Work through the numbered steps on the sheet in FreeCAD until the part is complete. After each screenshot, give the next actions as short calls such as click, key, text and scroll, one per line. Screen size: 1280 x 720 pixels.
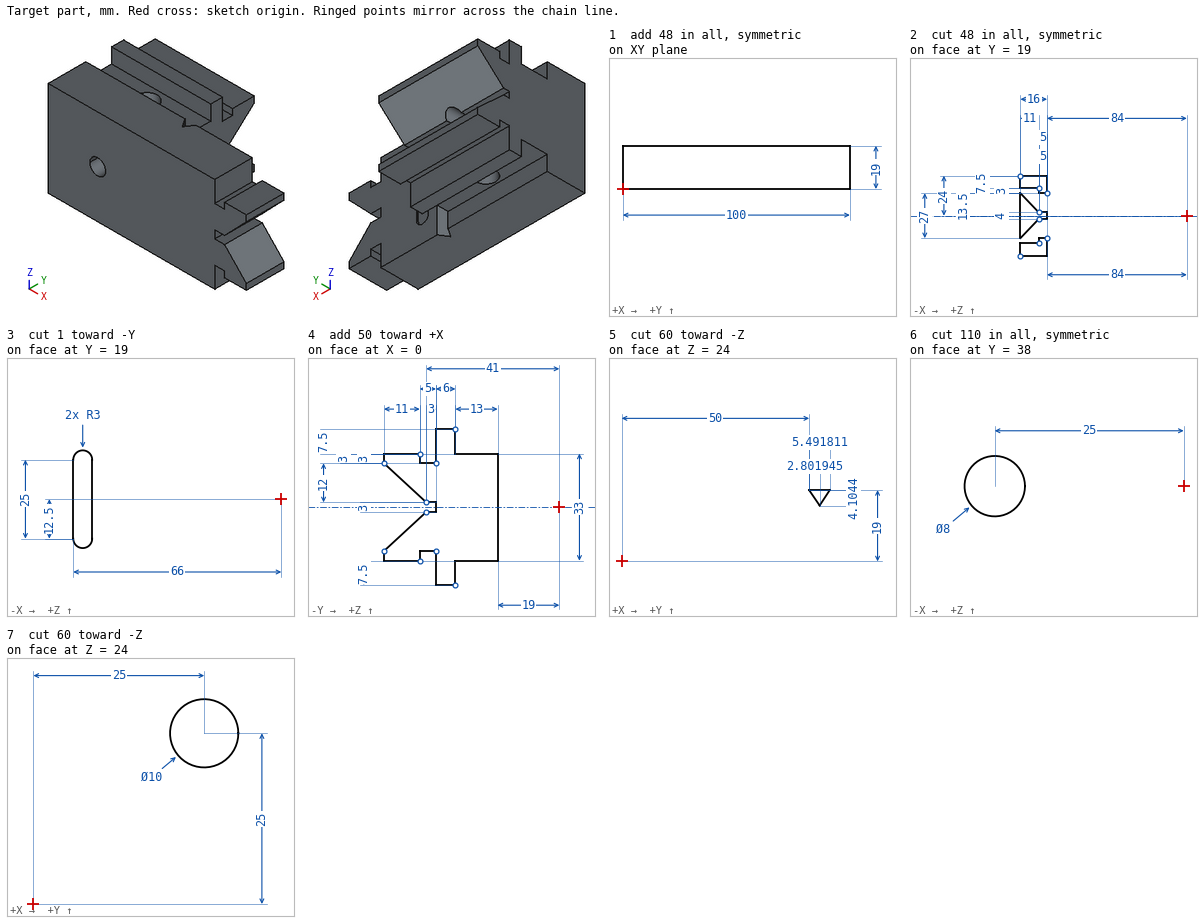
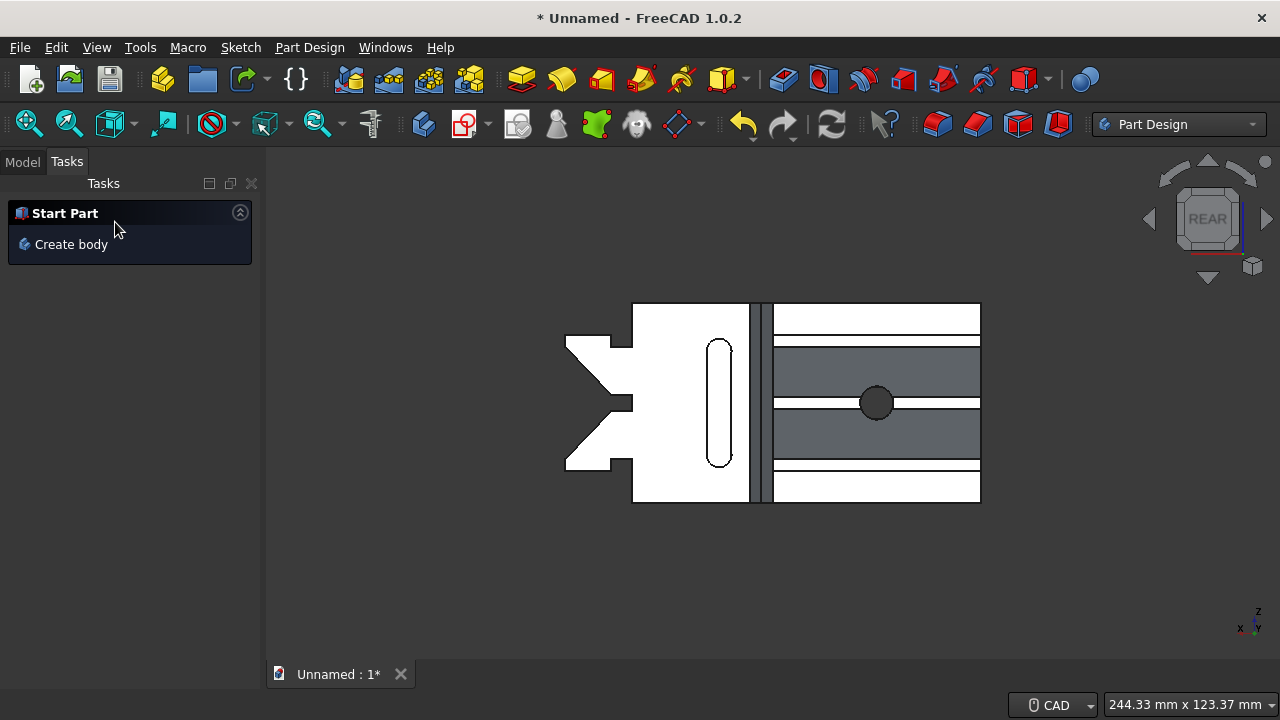
click(30, 124)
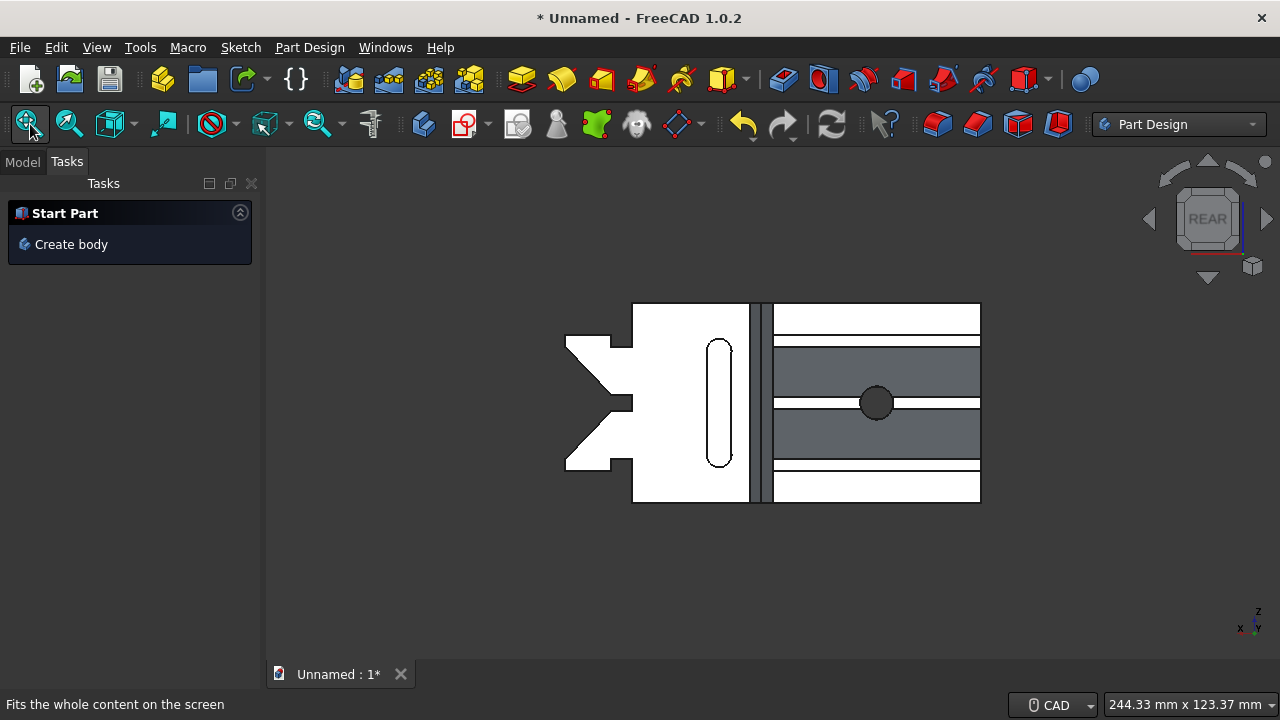
key(0)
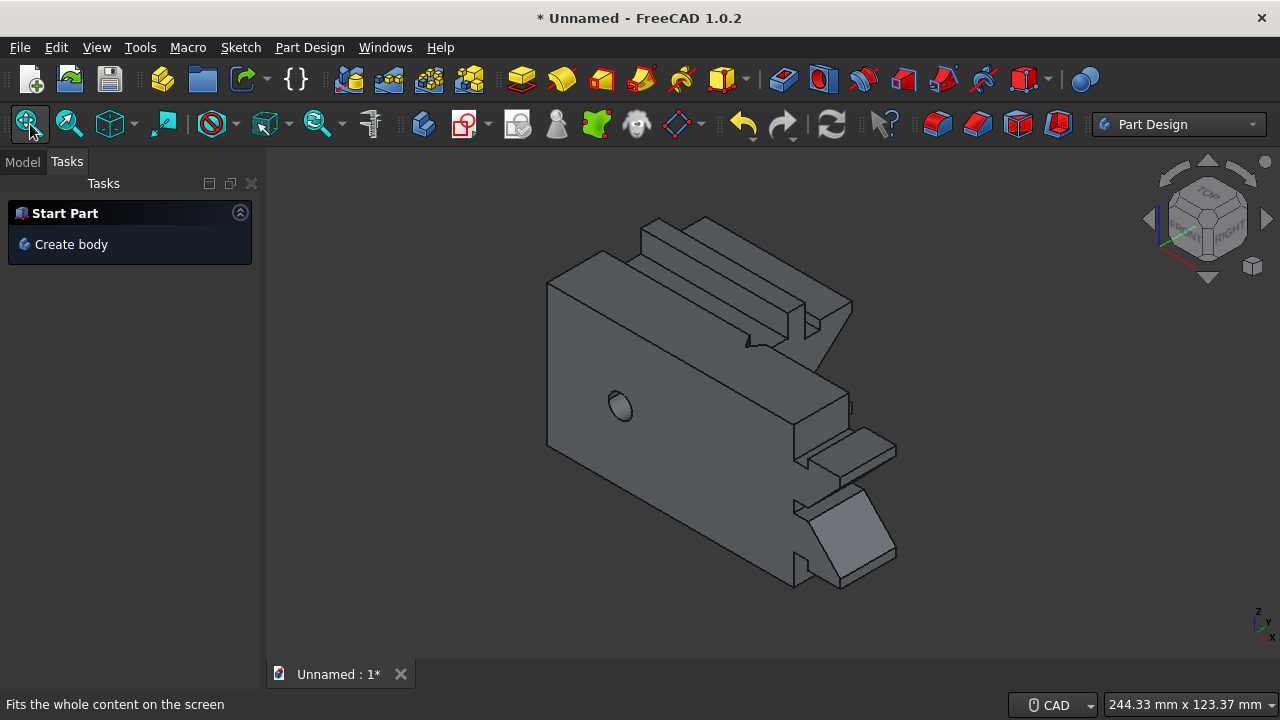
click(769, 377)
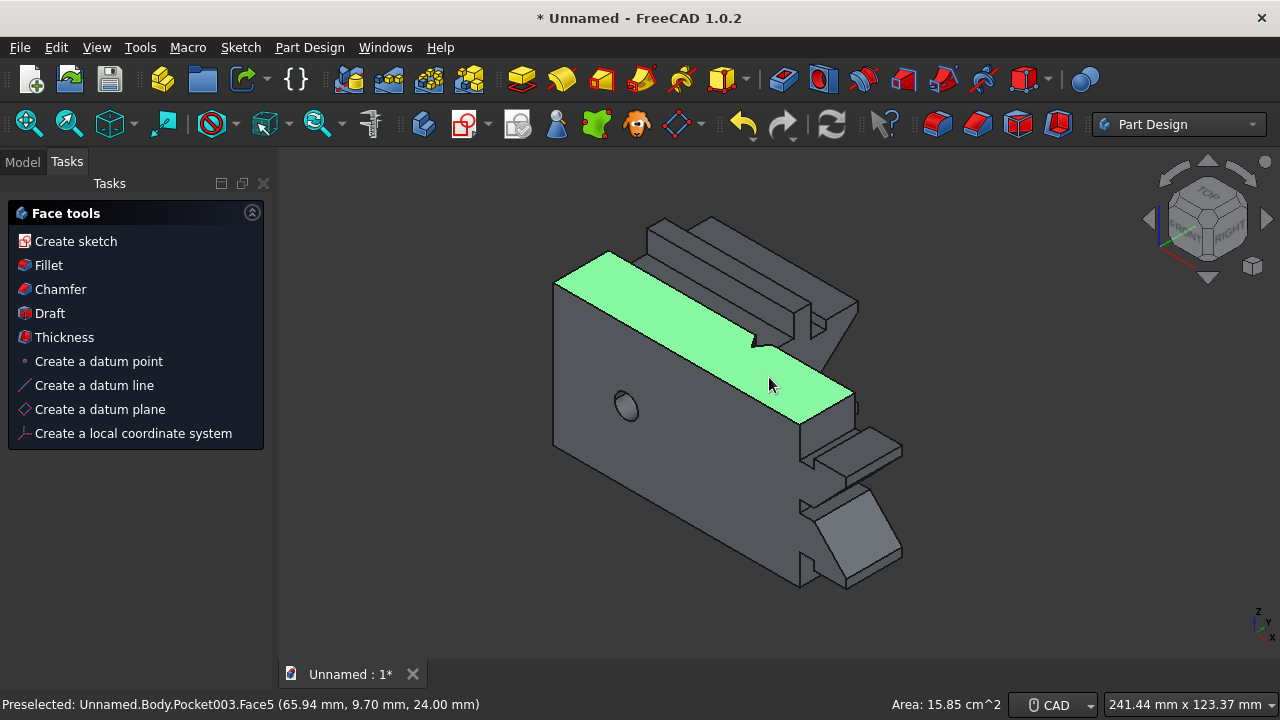
click(464, 124)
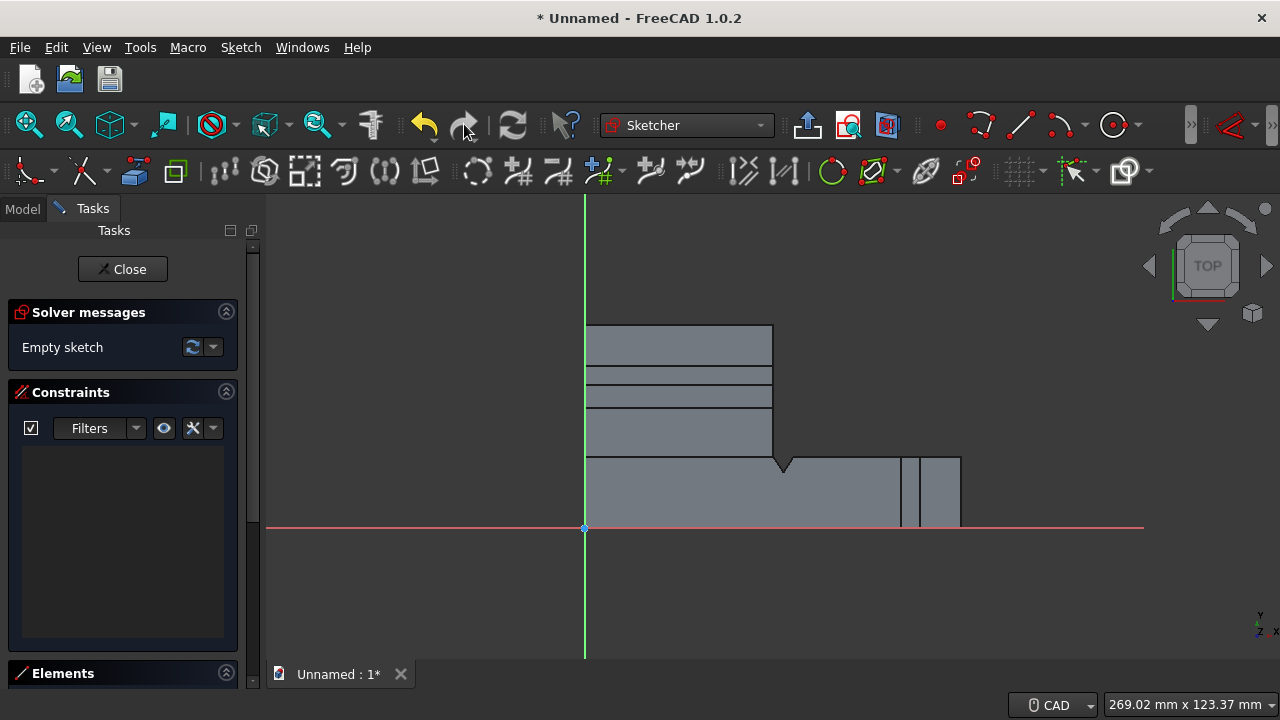
scroll(675, 435, up, 10)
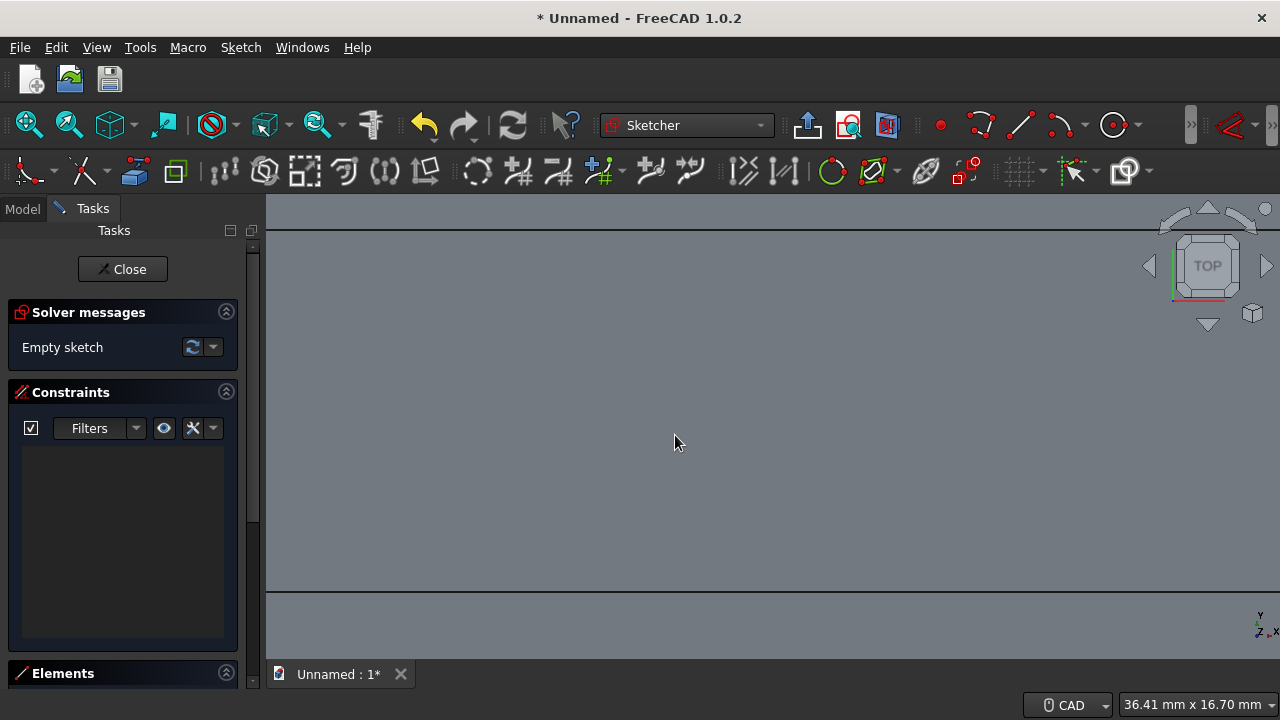
click(1114, 126)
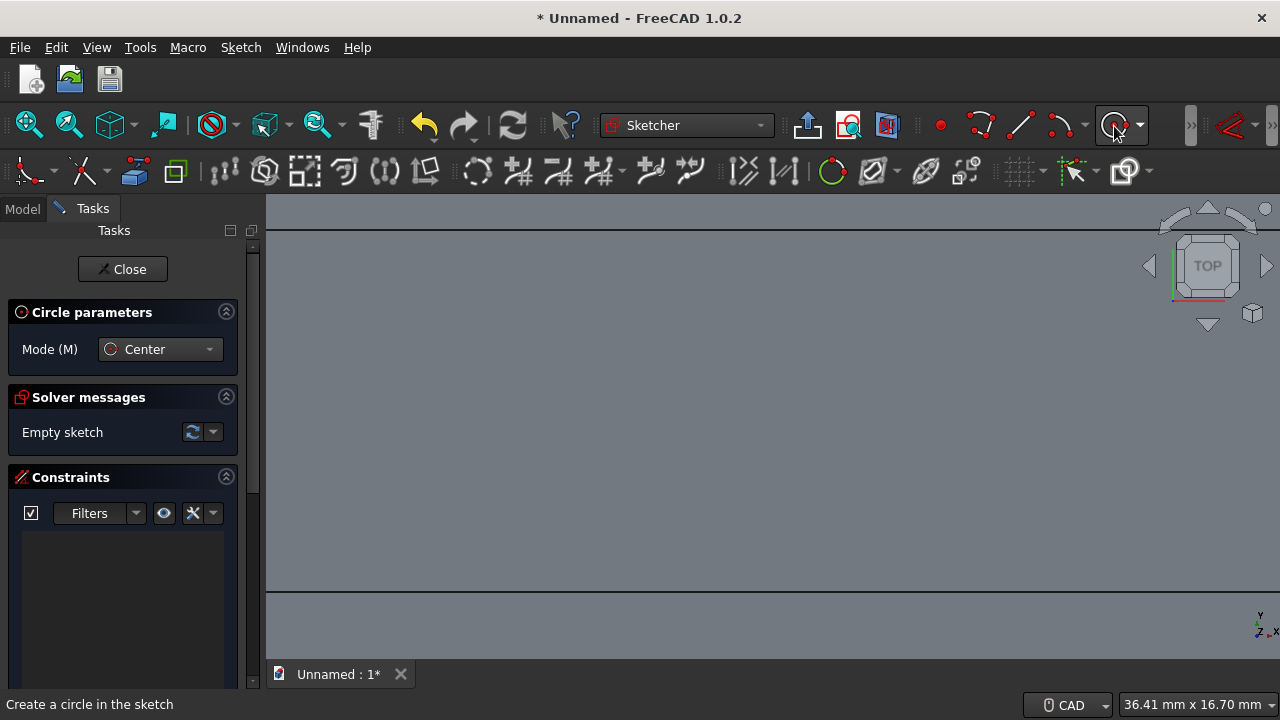
click(700, 425)
click(799, 326)
key(Escape)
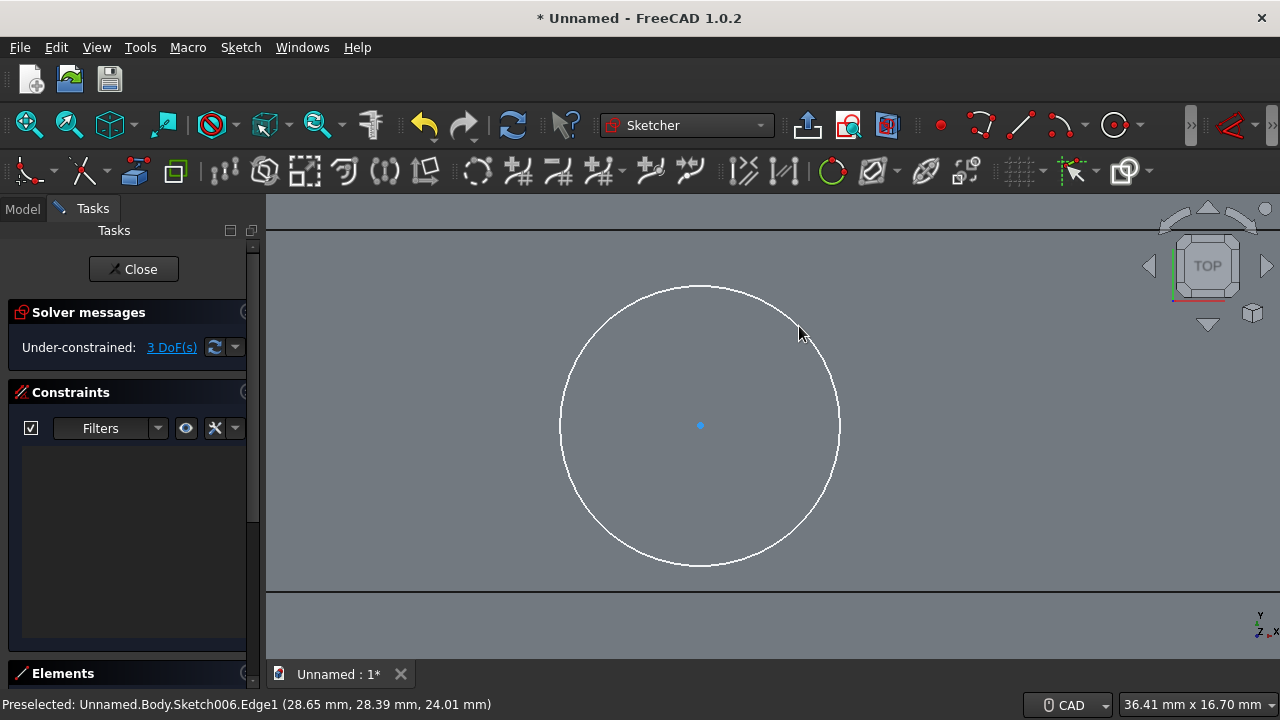
click(1230, 126)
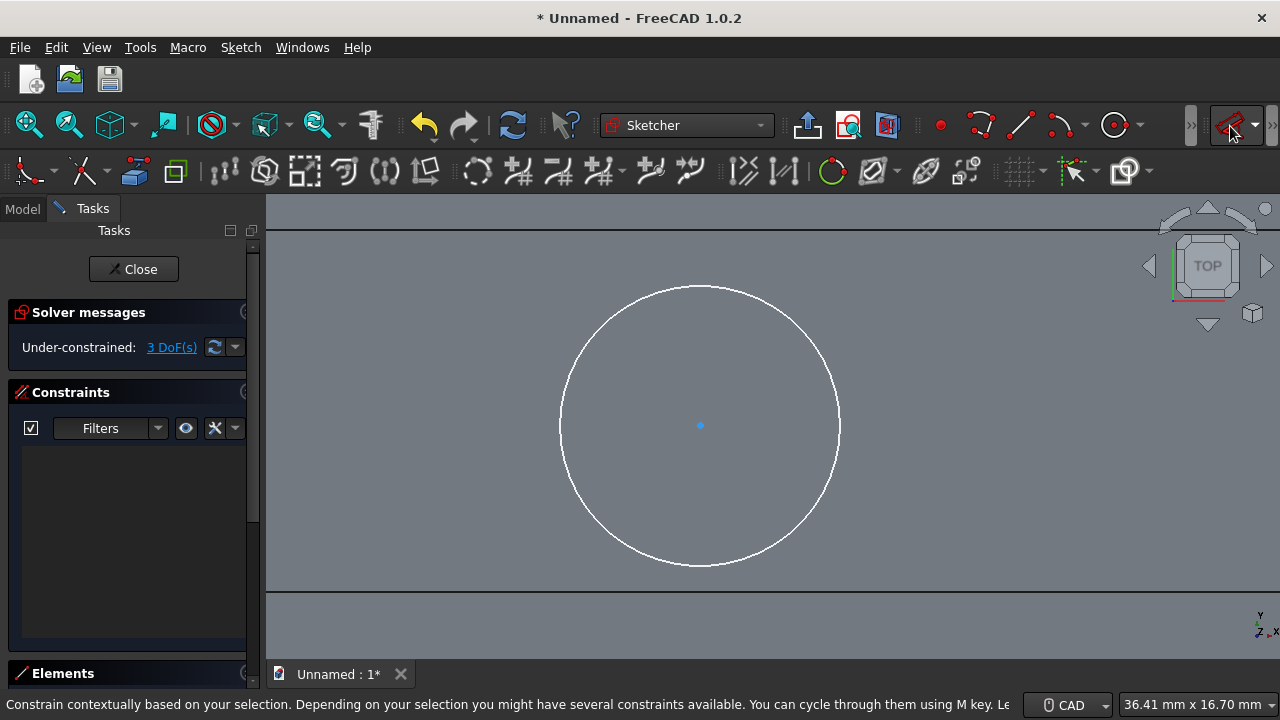
click(799, 327)
click(822, 304)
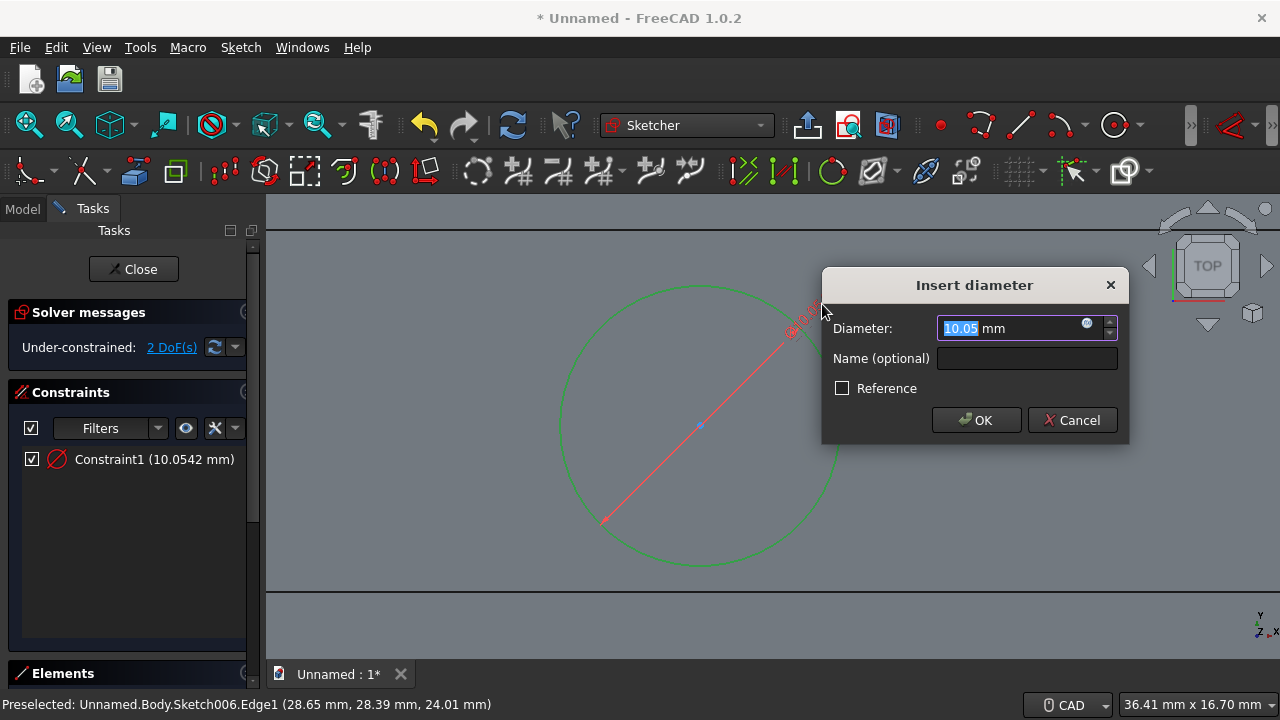
text(10)
key(Return)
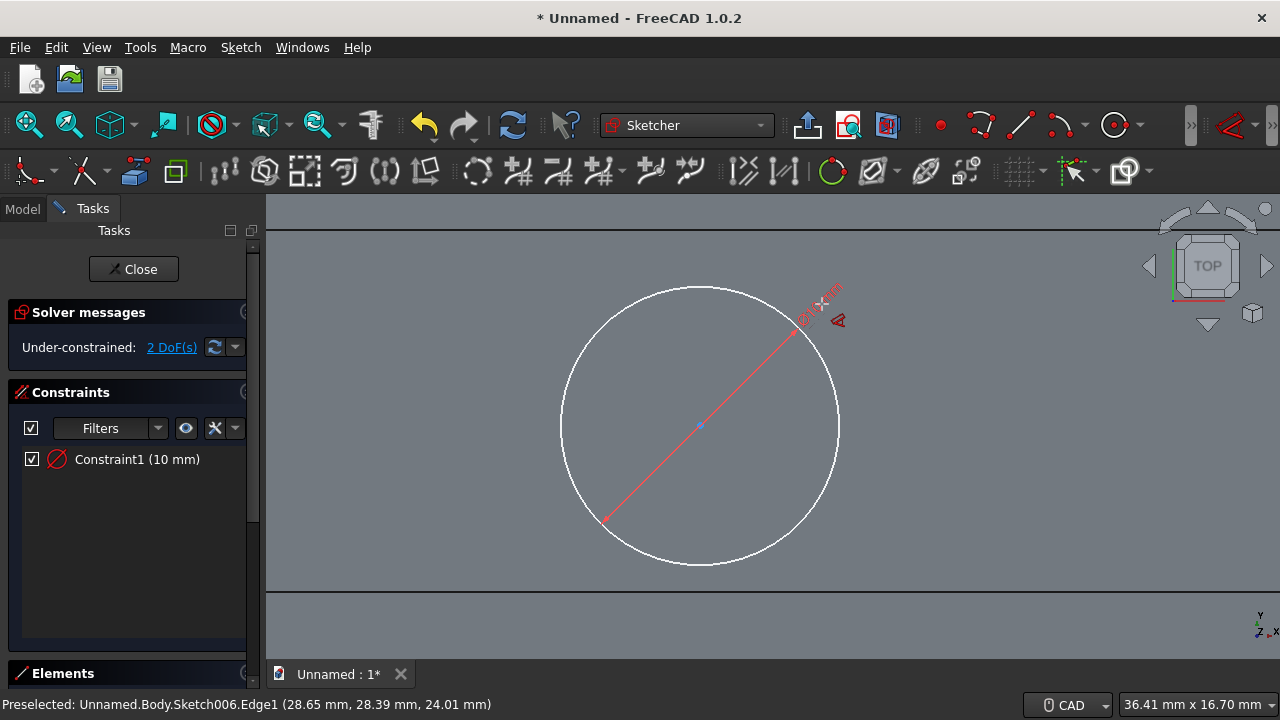
click(700, 426)
click(497, 392)